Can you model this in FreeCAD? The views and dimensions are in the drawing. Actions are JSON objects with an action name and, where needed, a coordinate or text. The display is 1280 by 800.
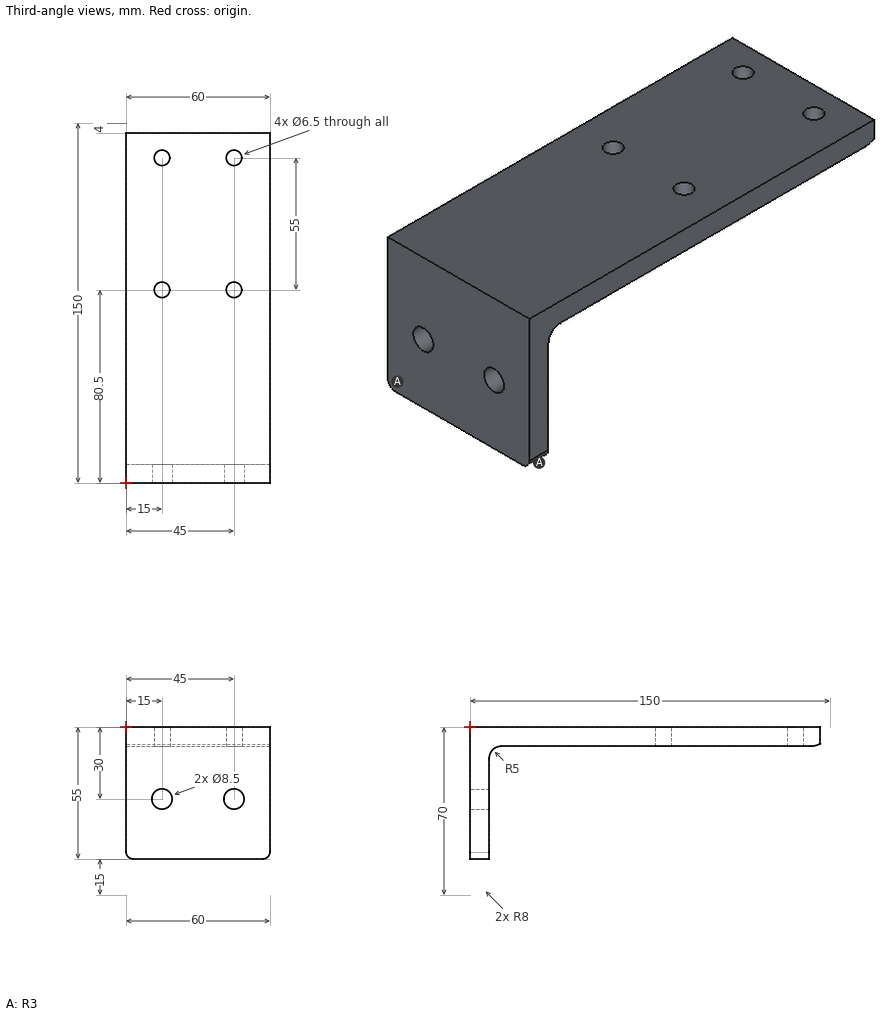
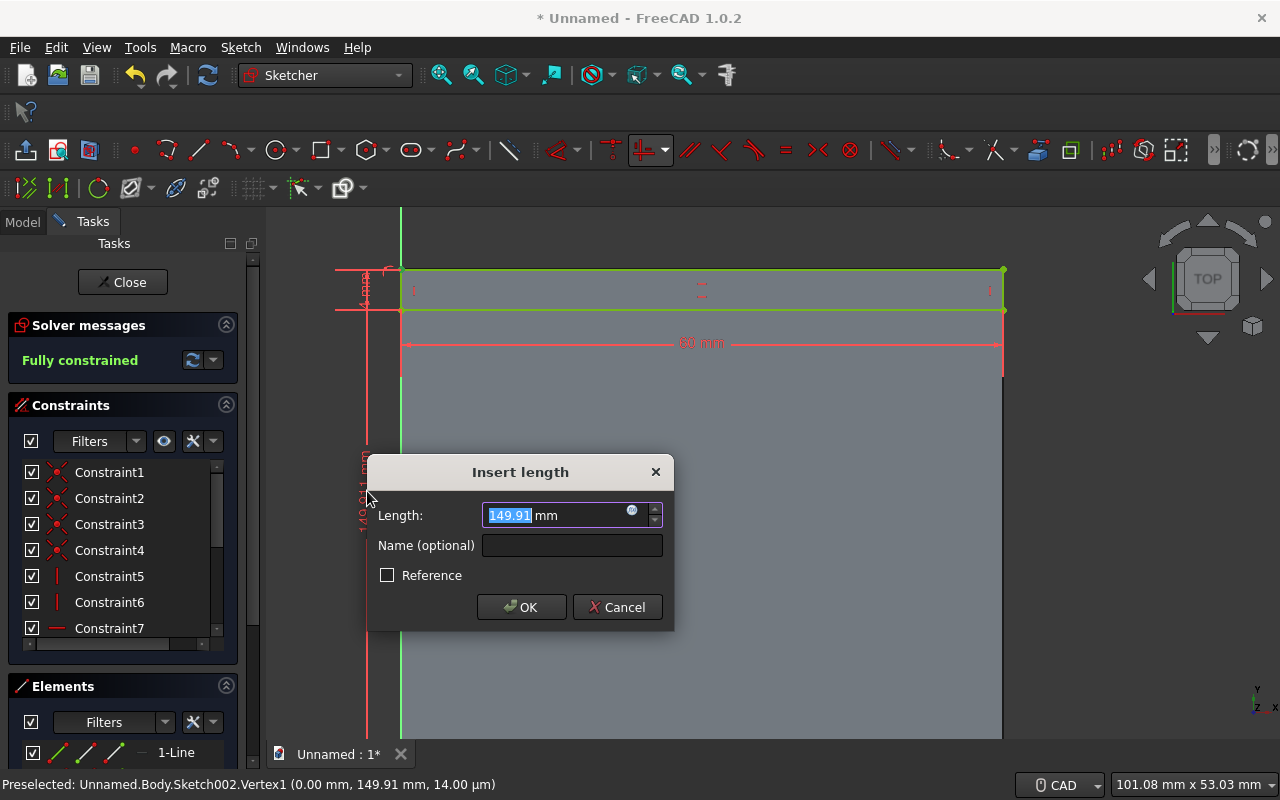
{"action": "type", "text": "150"}
{"action": "key", "text": "Return"}
{"action": "key", "text": "Escape"}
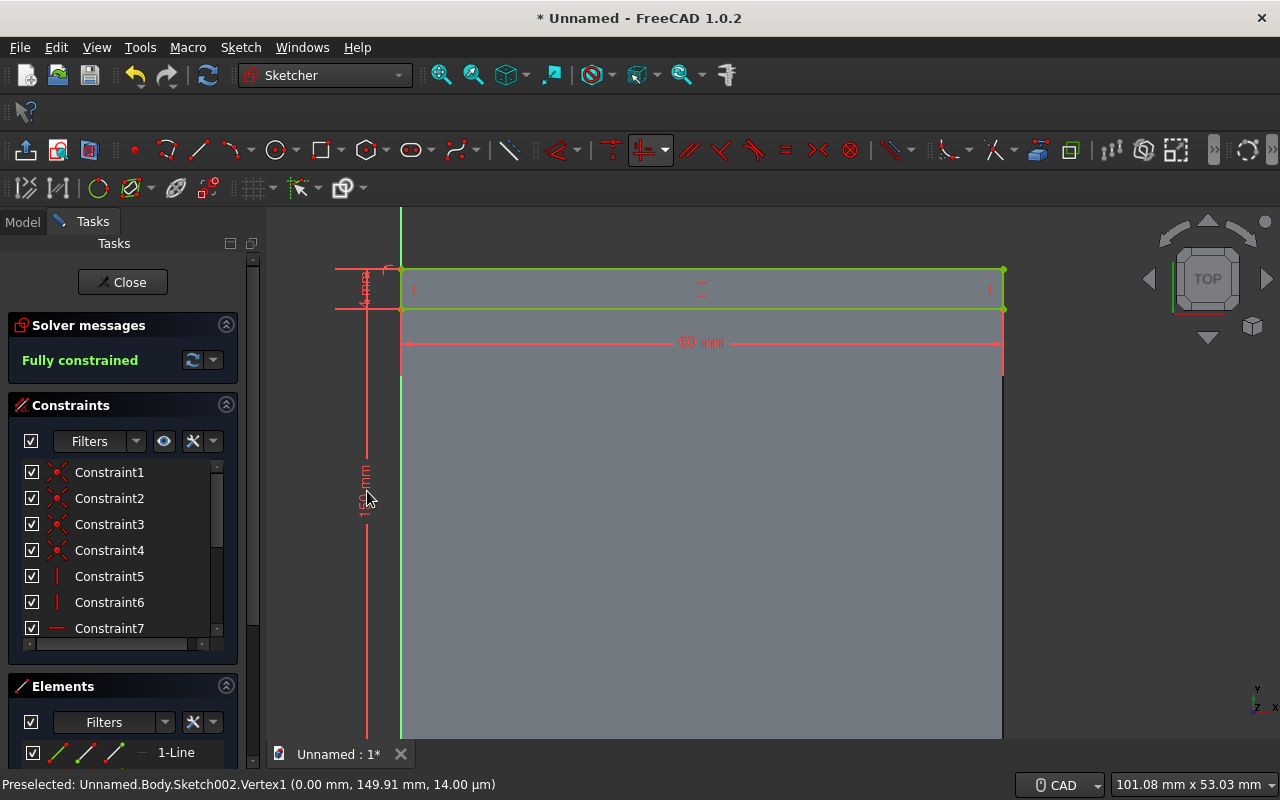
{"action": "left_click", "coordinate": [123, 282]}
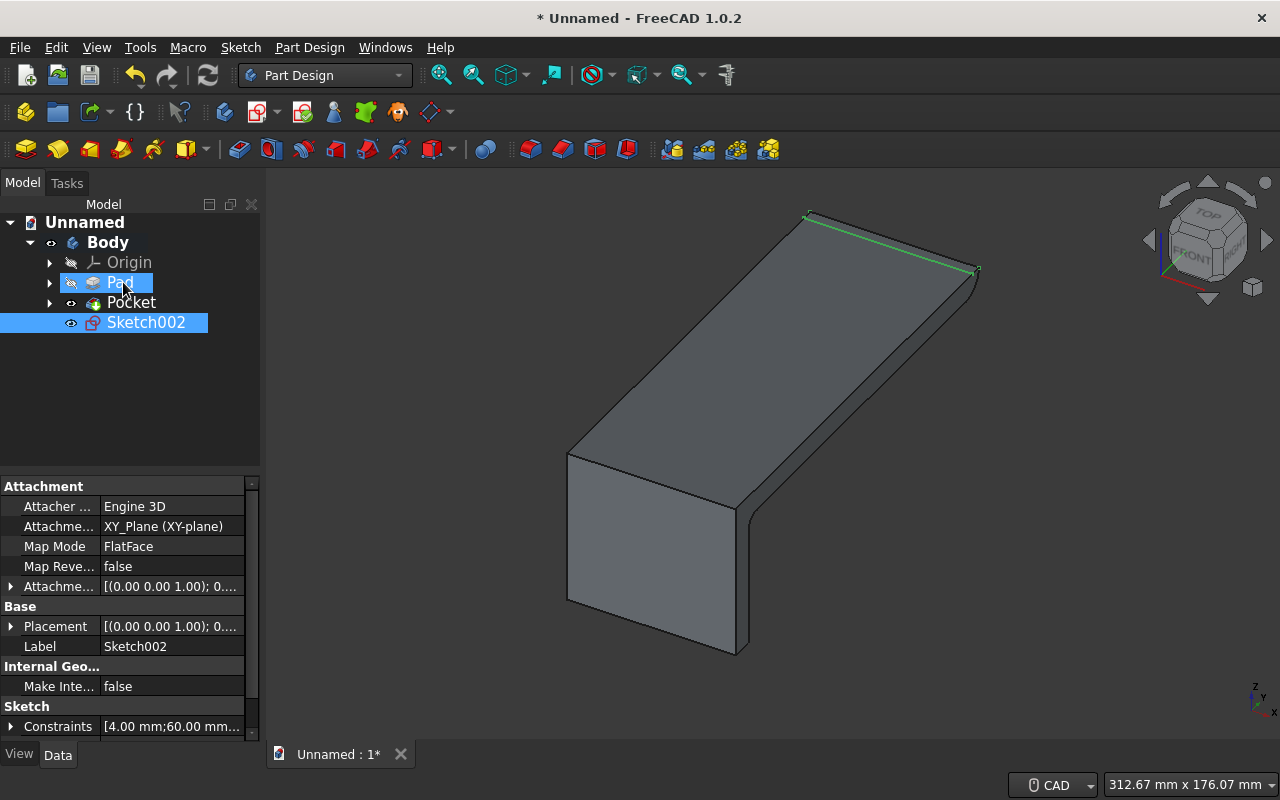
{"action": "left_click", "coordinate": [240, 150]}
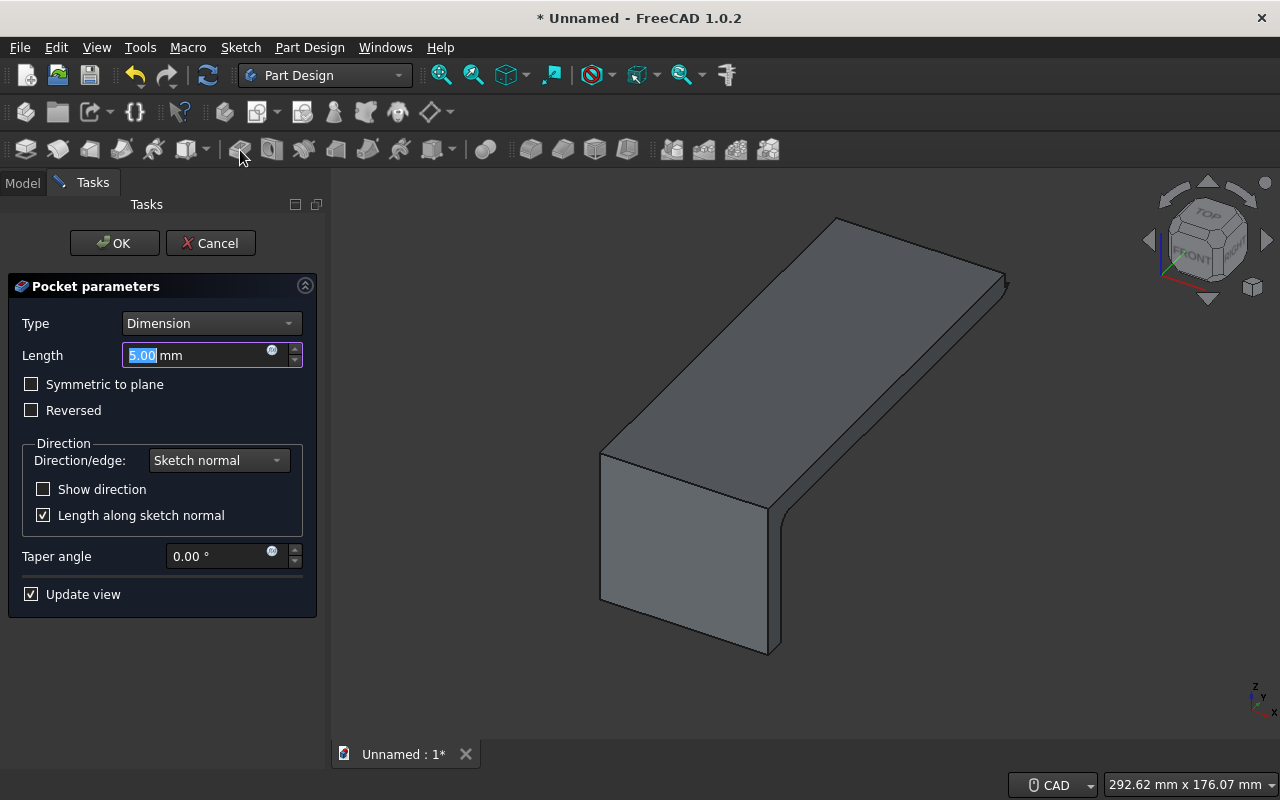
{"action": "left_click", "coordinate": [212, 324]}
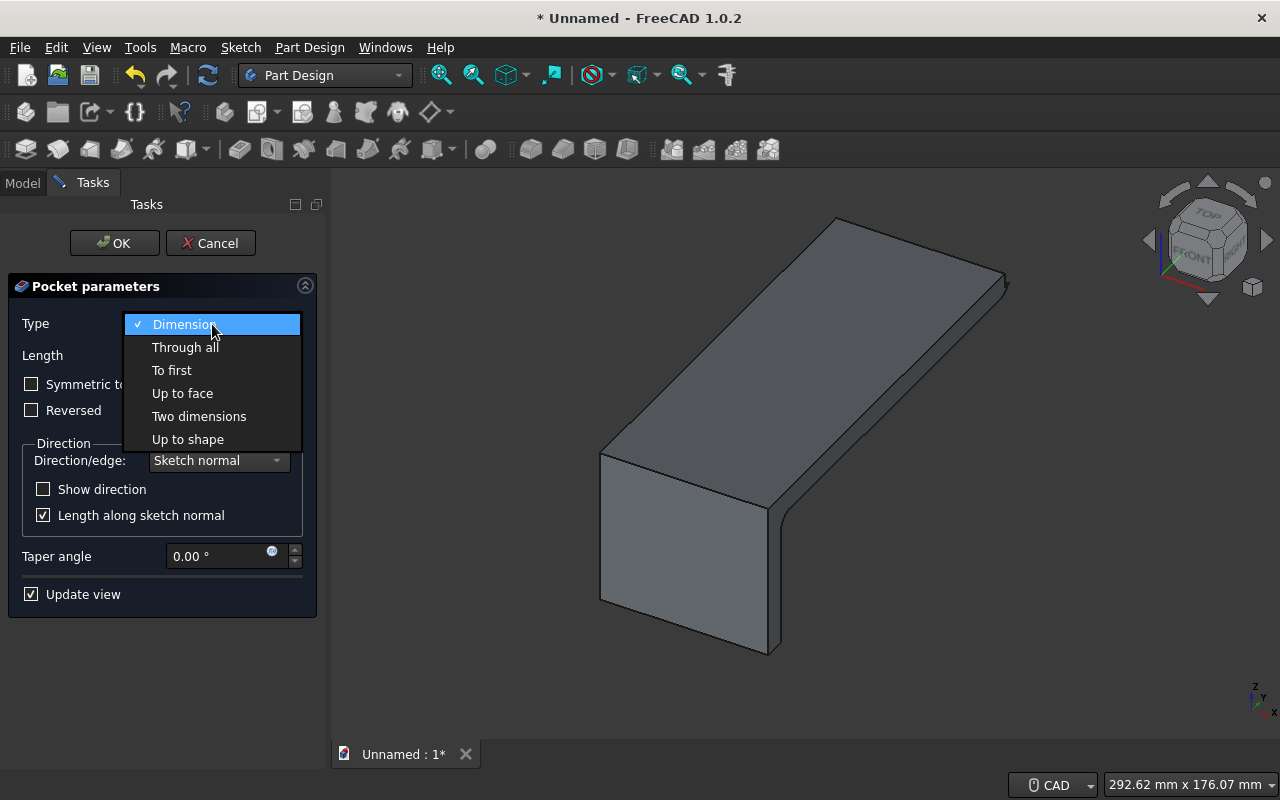
{"action": "left_click", "coordinate": [212, 348]}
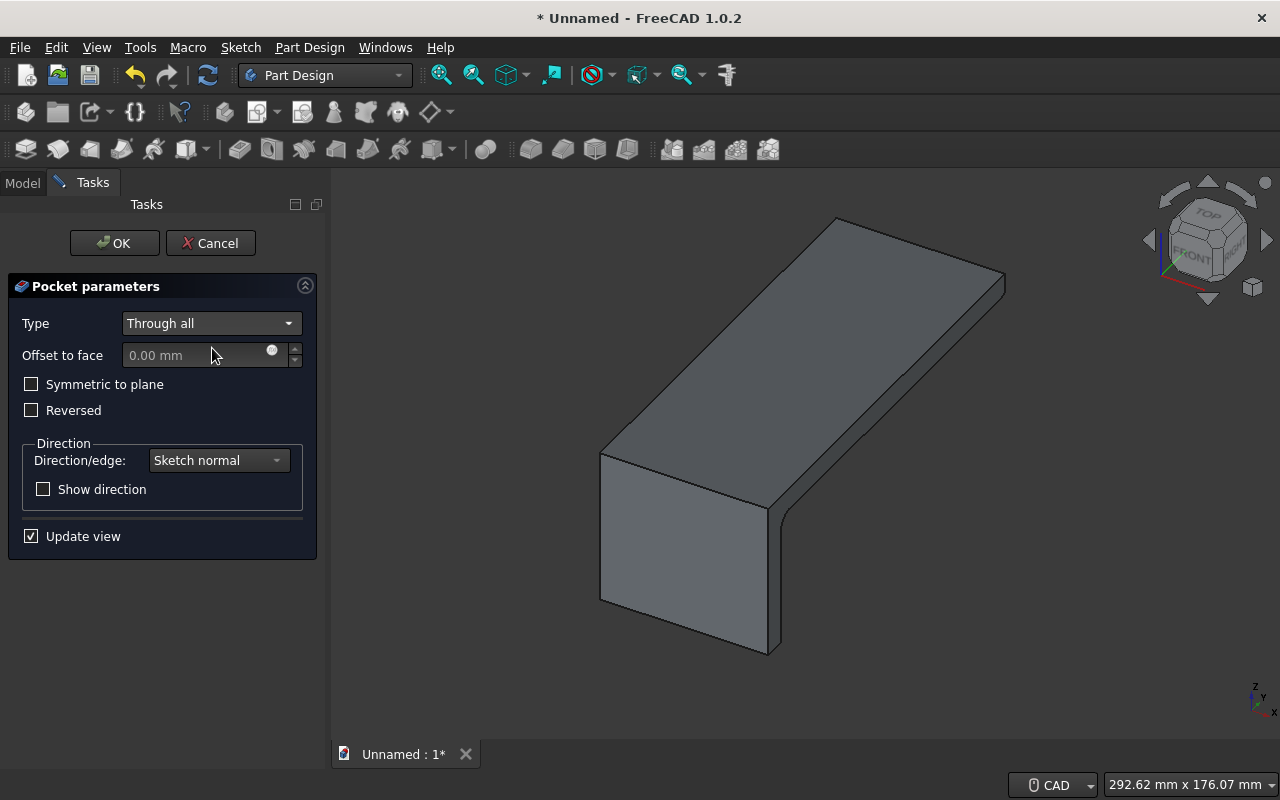
{"action": "left_click", "coordinate": [115, 243]}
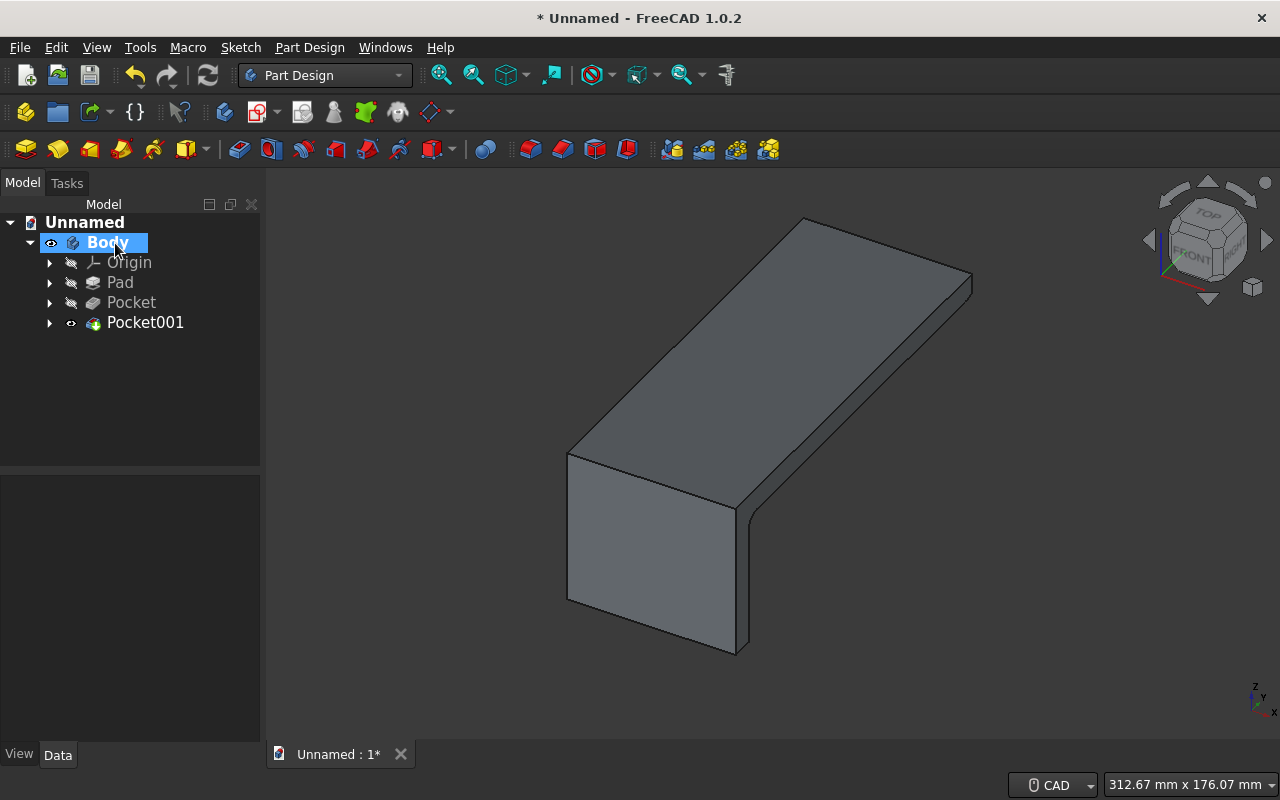
{"action": "key", "text": "5"}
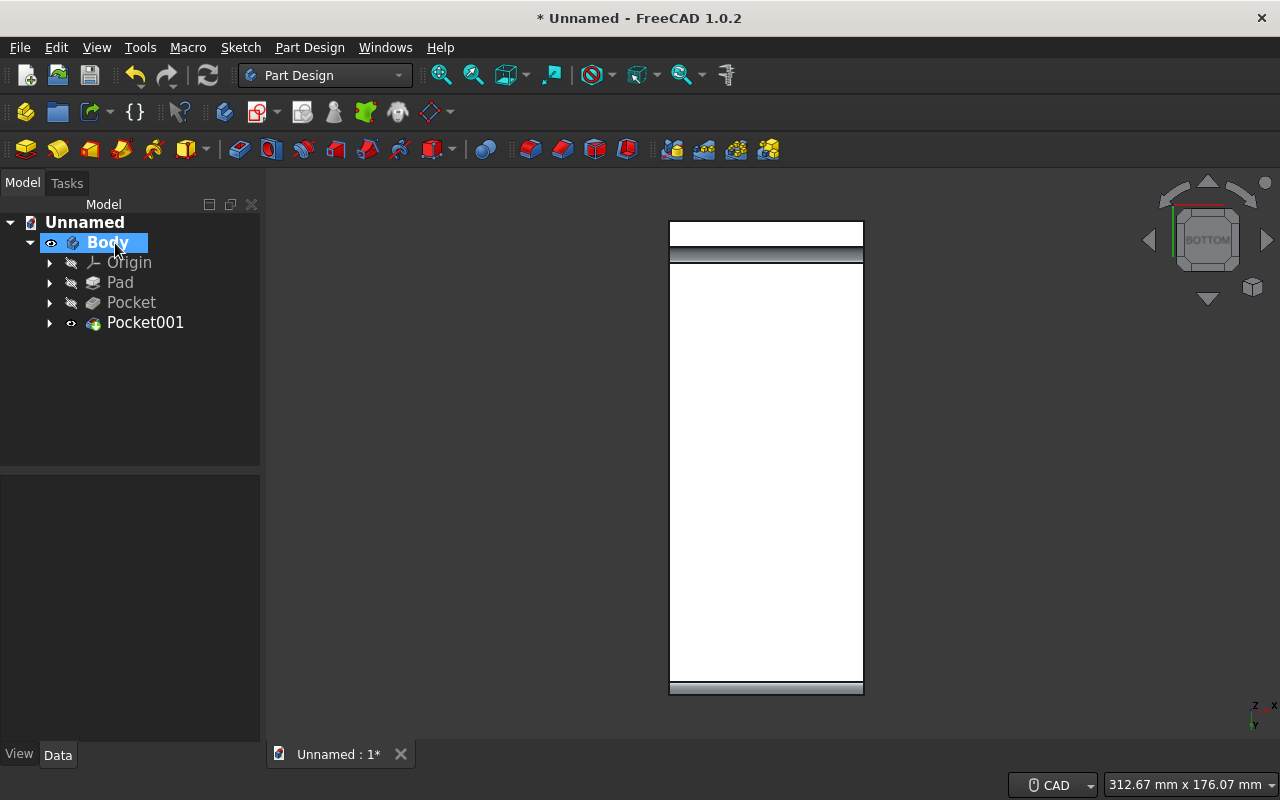
{"action": "left_click", "coordinate": [767, 531]}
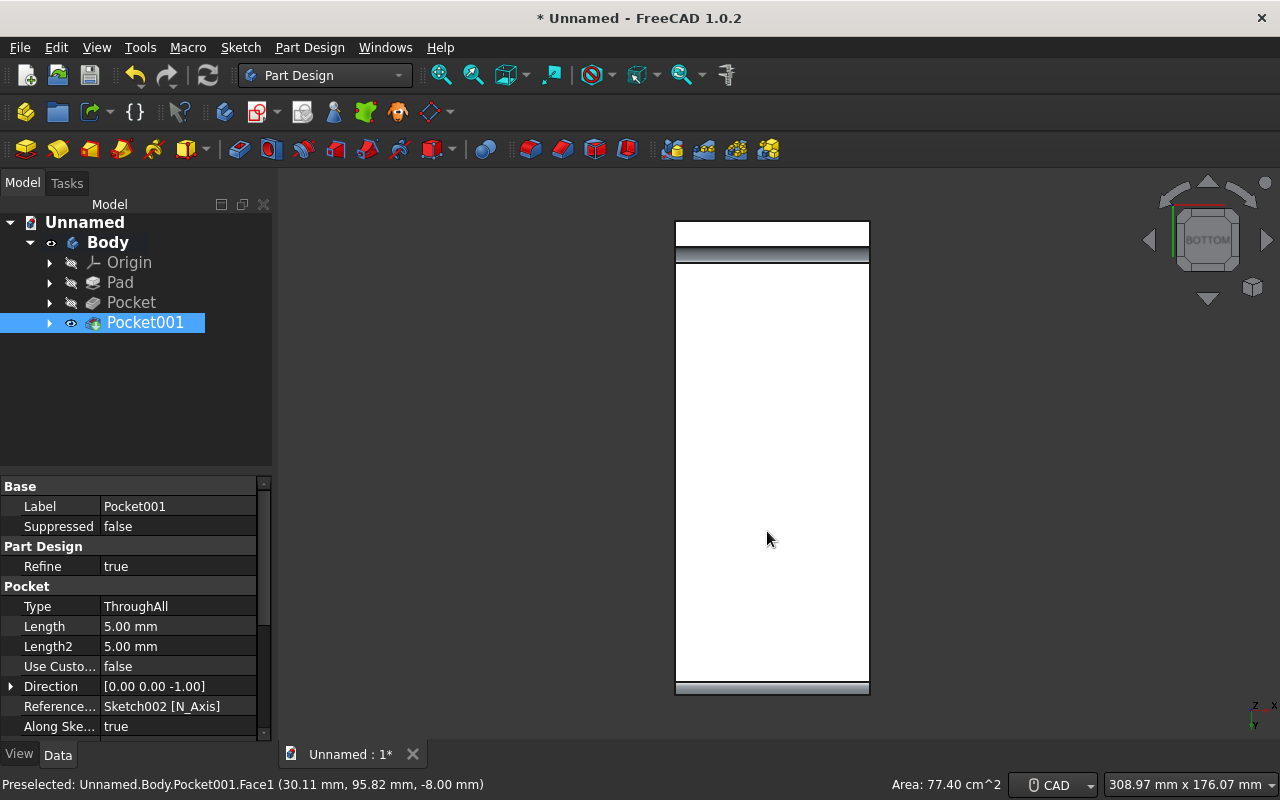
{"action": "left_click", "coordinate": [258, 112]}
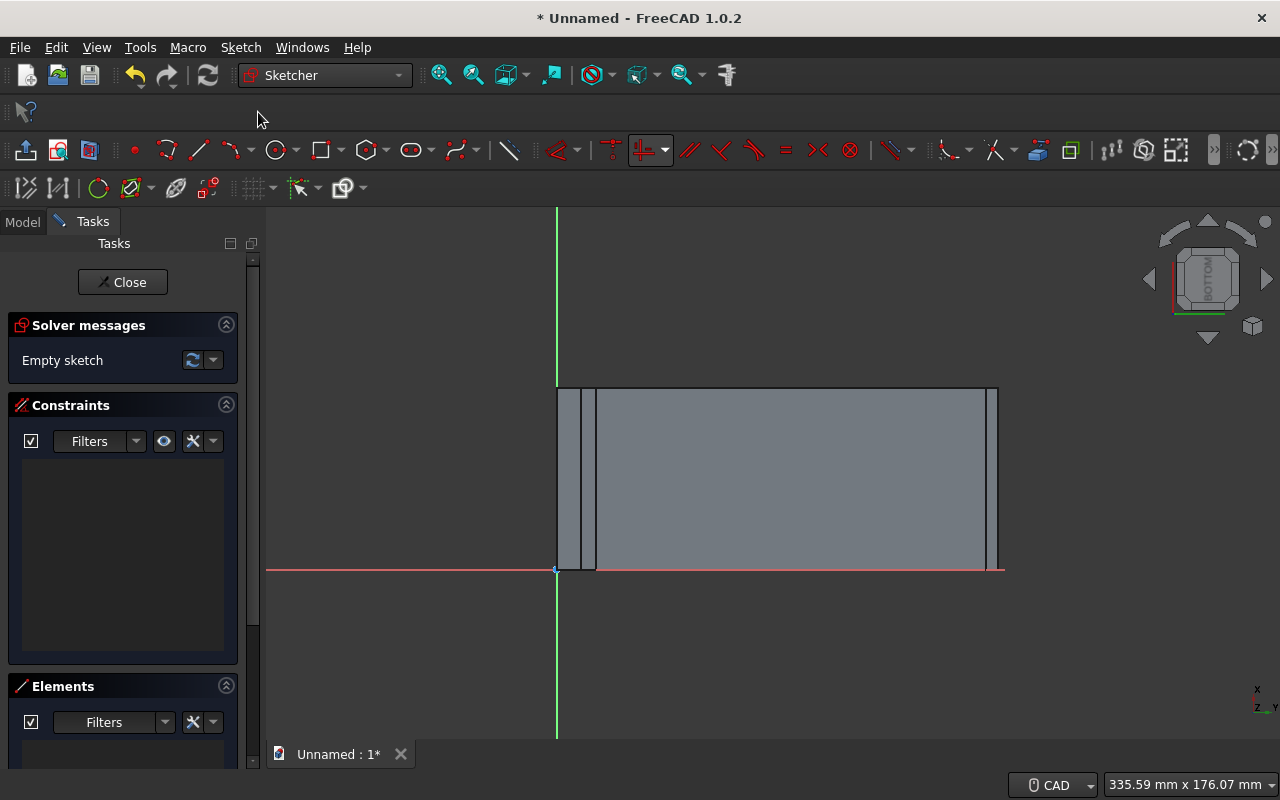
{"action": "scroll", "coordinate": [892, 545], "scroll_direction": "up", "scroll_amount": 2}